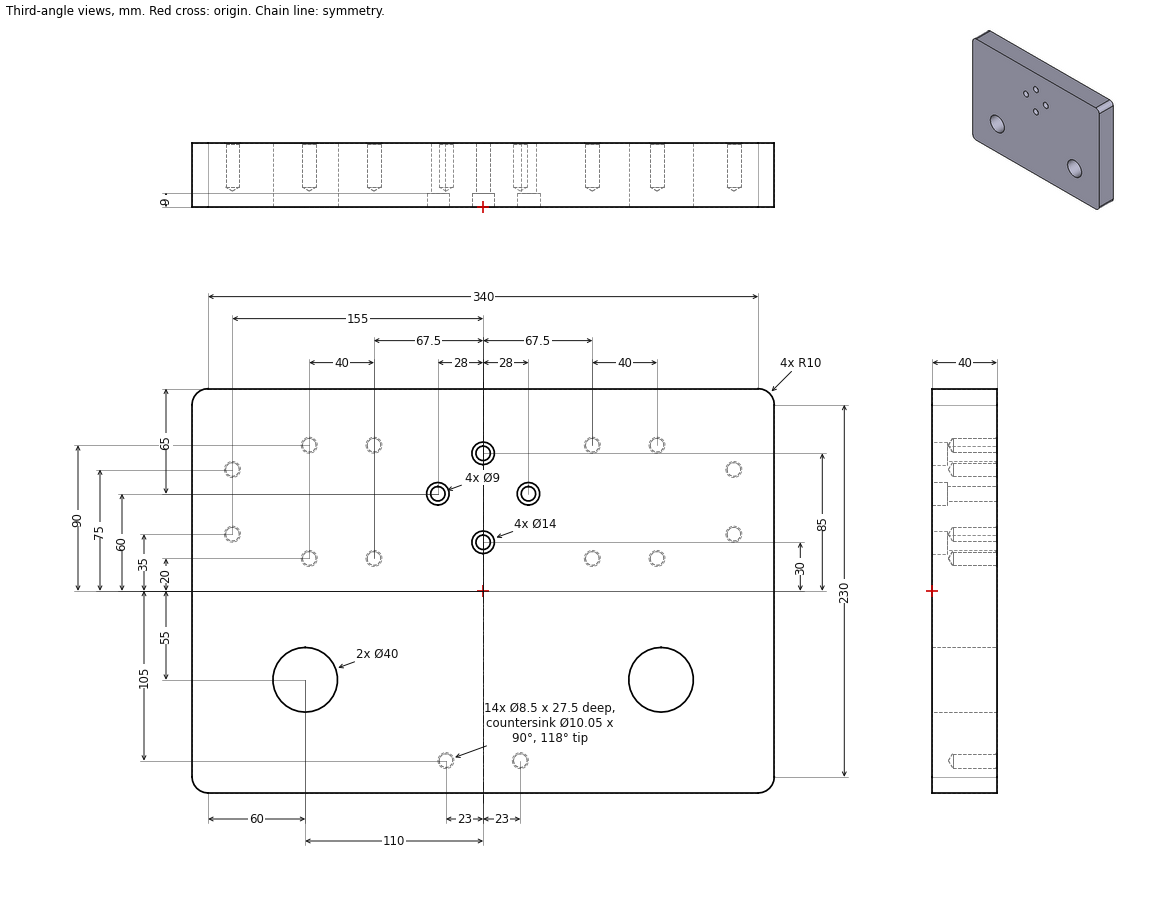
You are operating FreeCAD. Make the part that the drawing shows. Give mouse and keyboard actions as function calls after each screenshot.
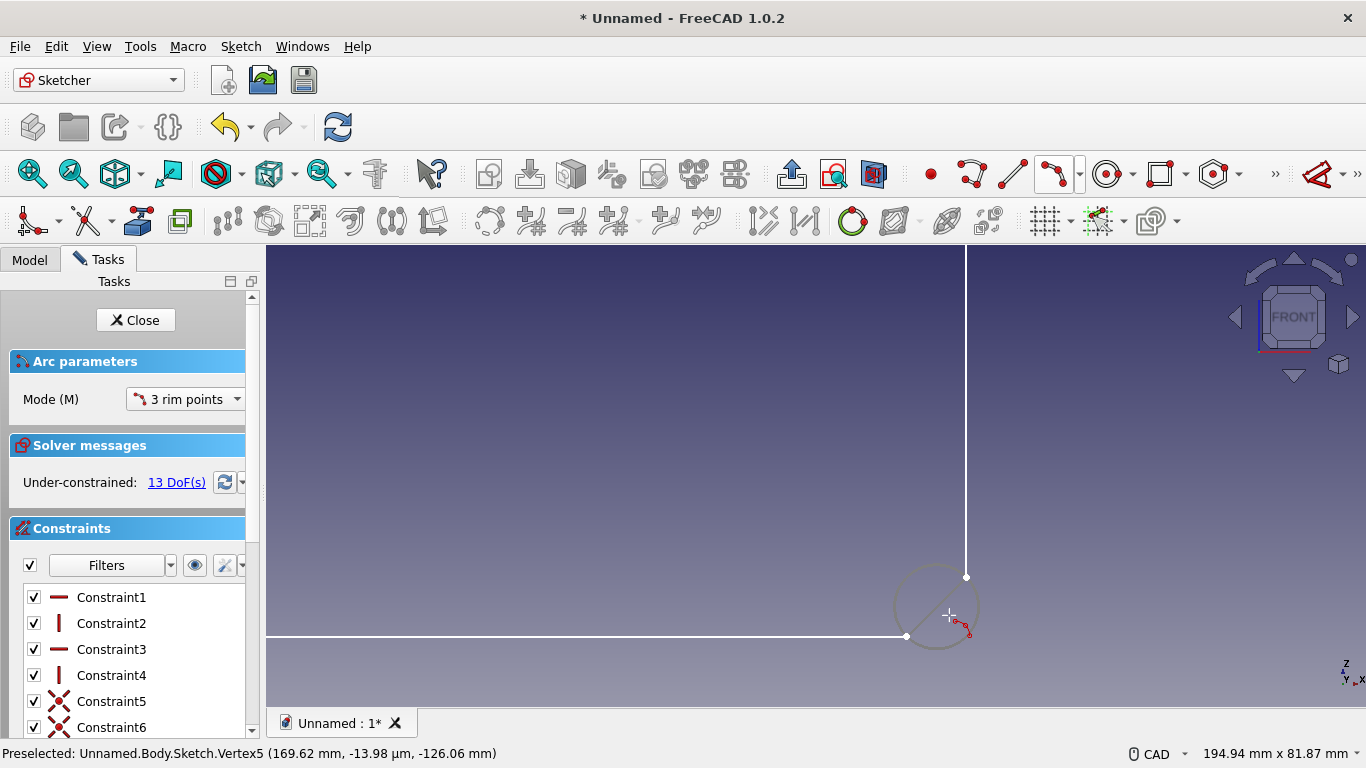
click(949, 614)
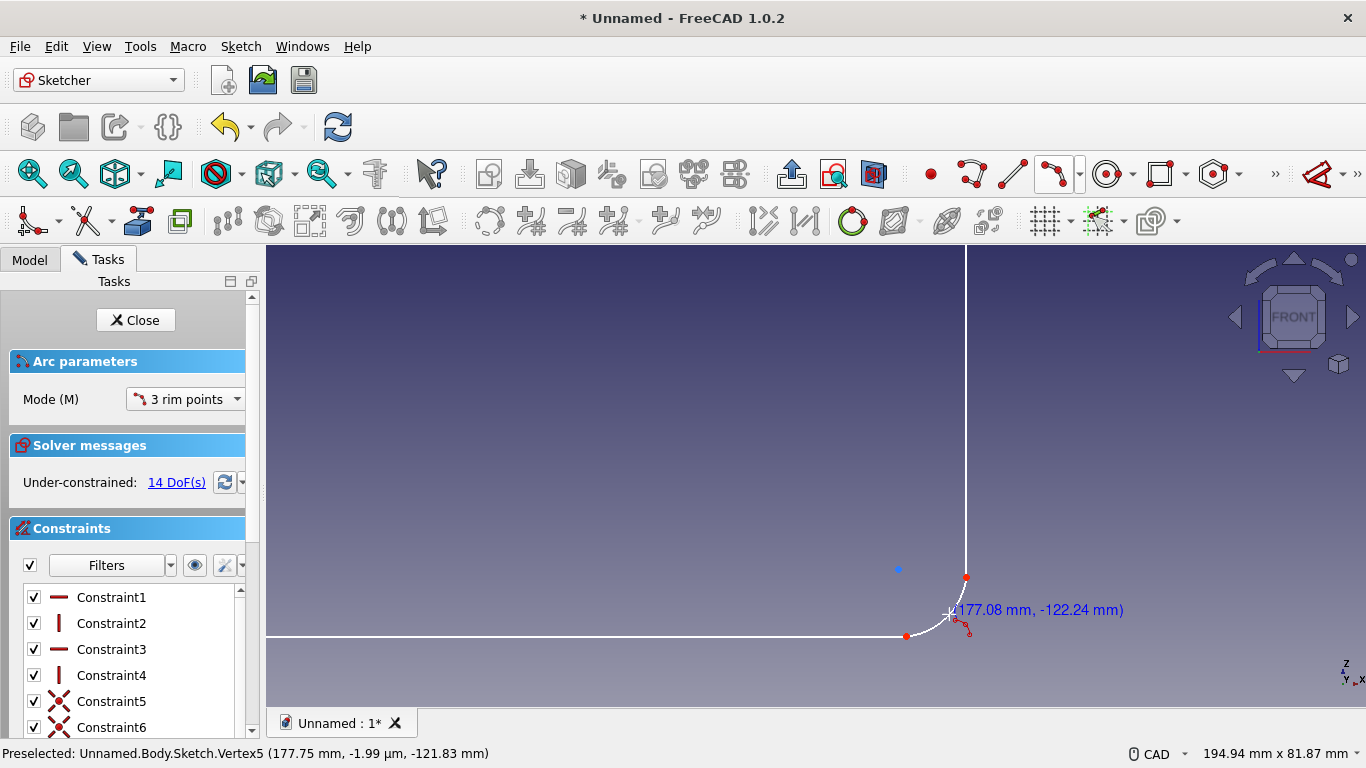
scroll(949, 615, down, 8)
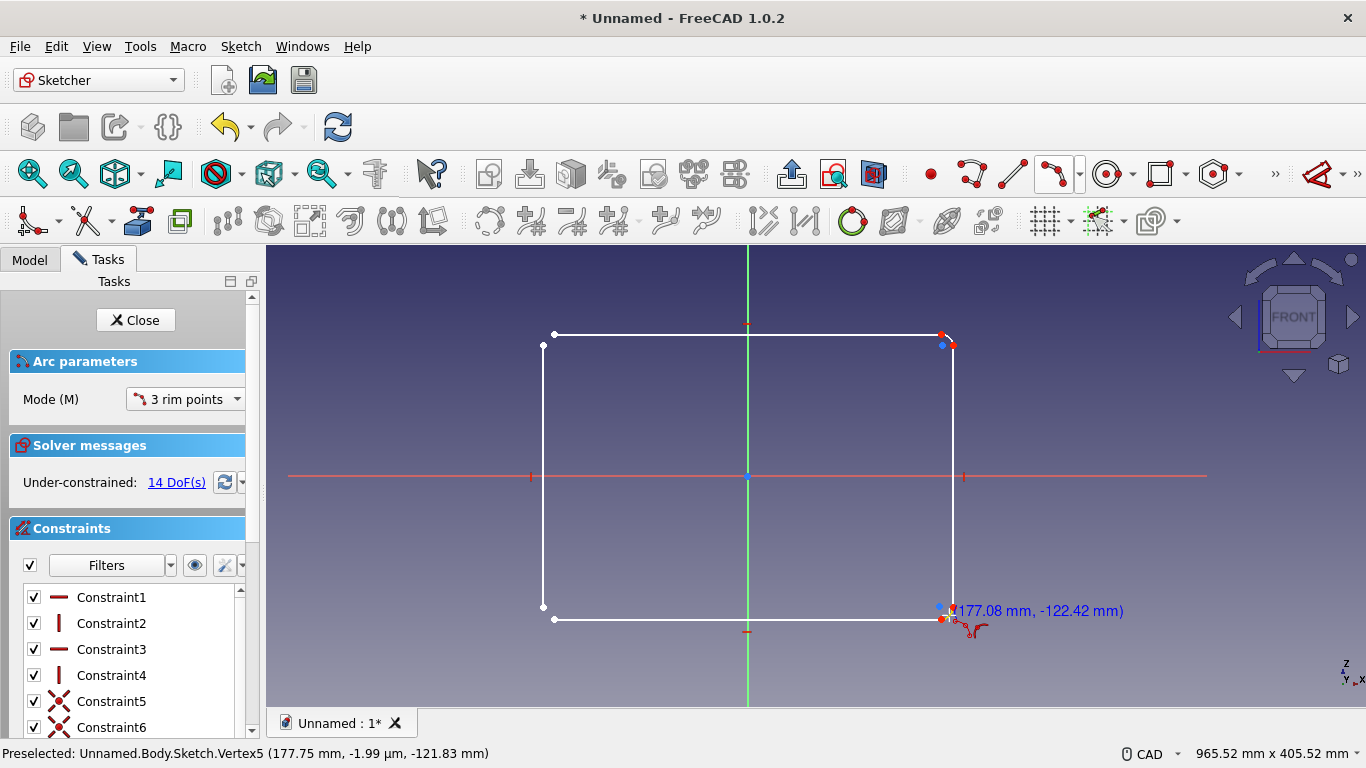
click(554, 620)
click(543, 608)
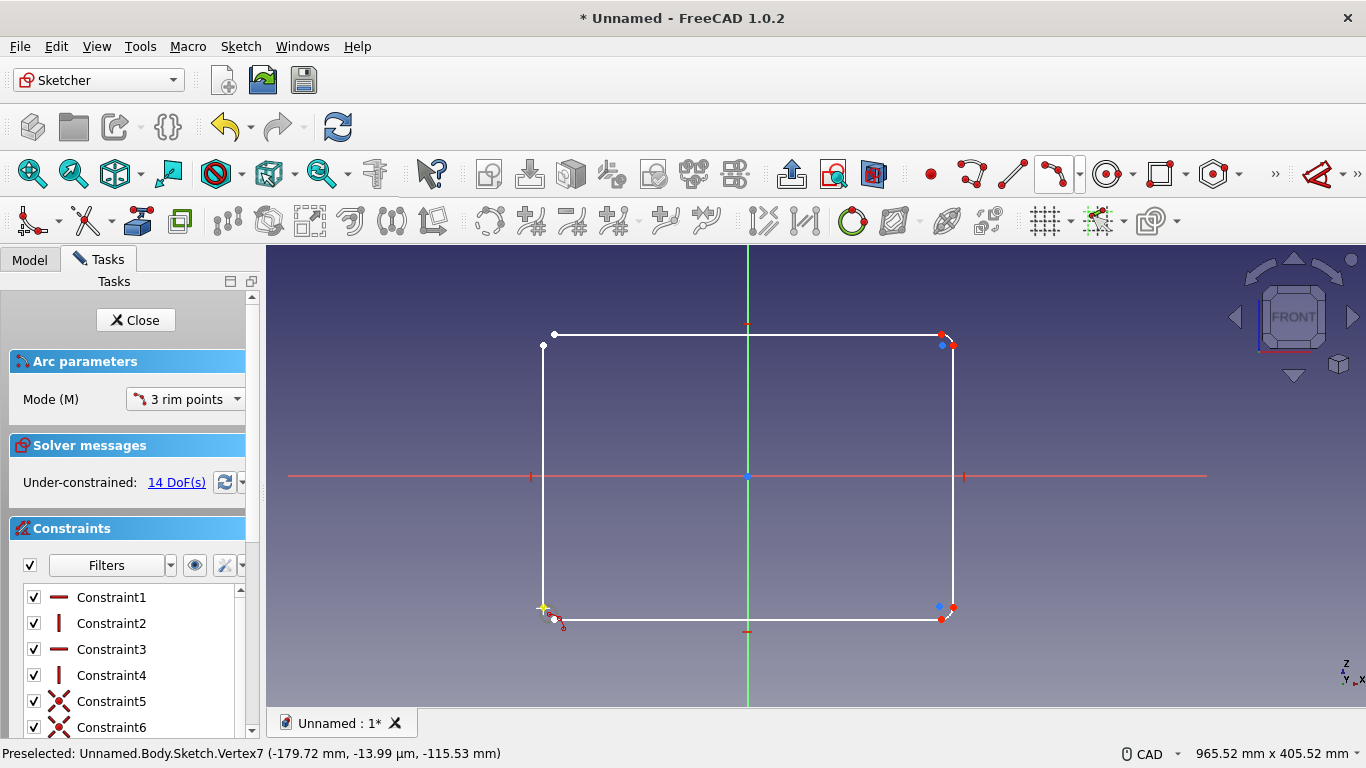
scroll(546, 615, up, 8)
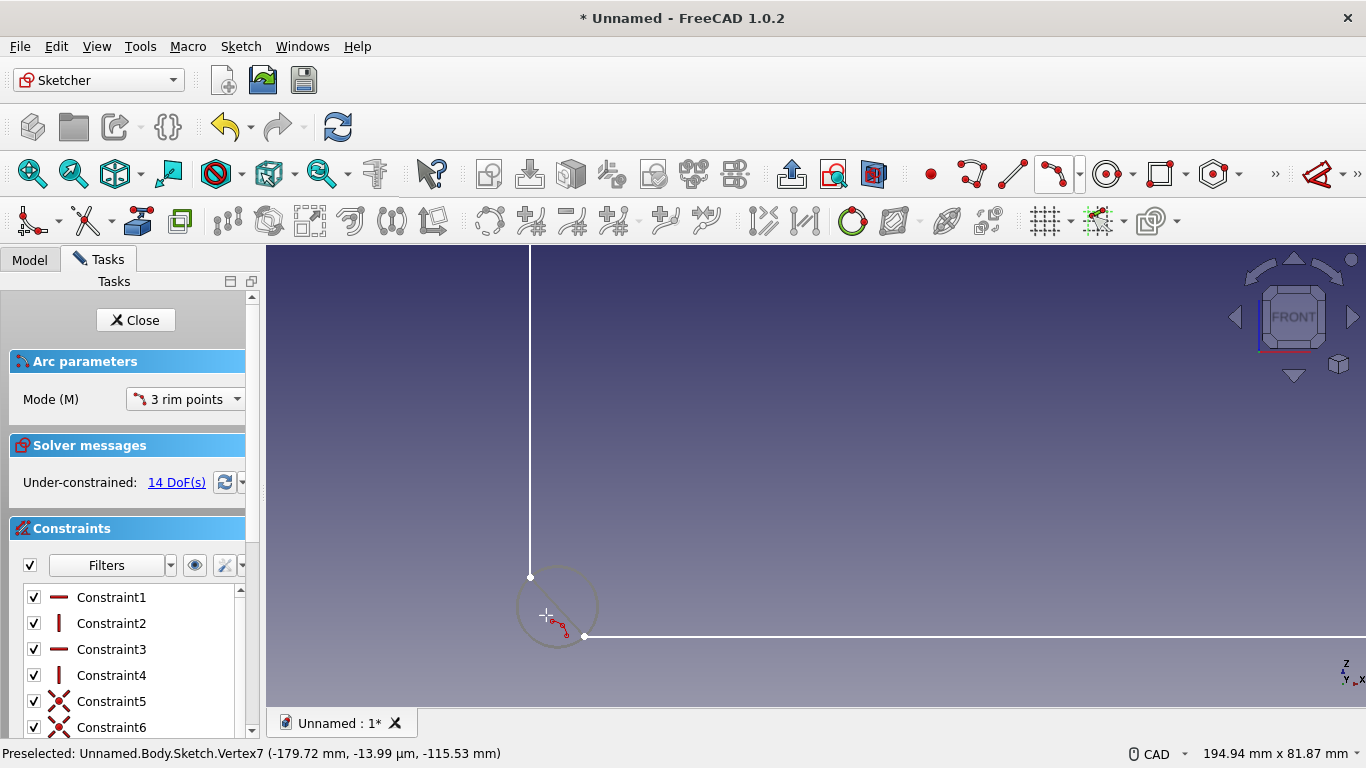
click(545, 614)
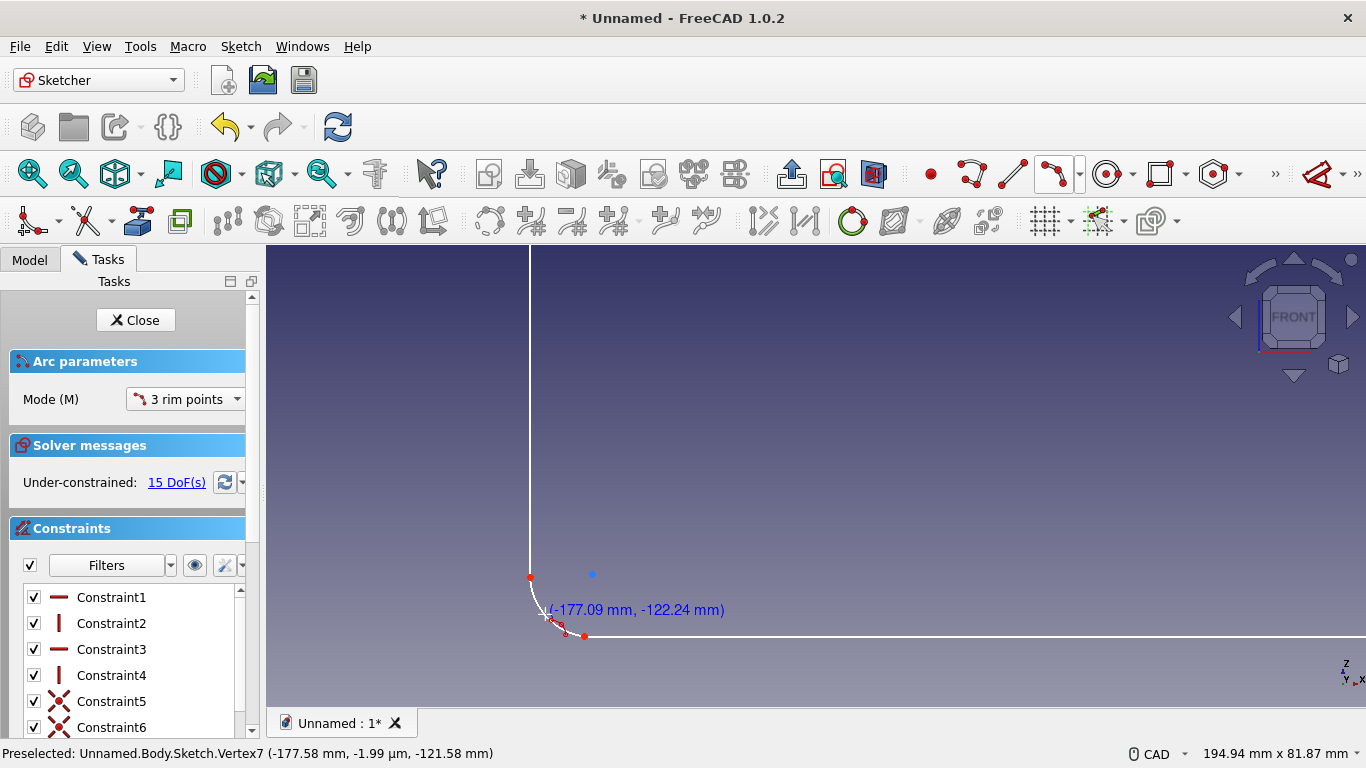
scroll(546, 615, down, 8)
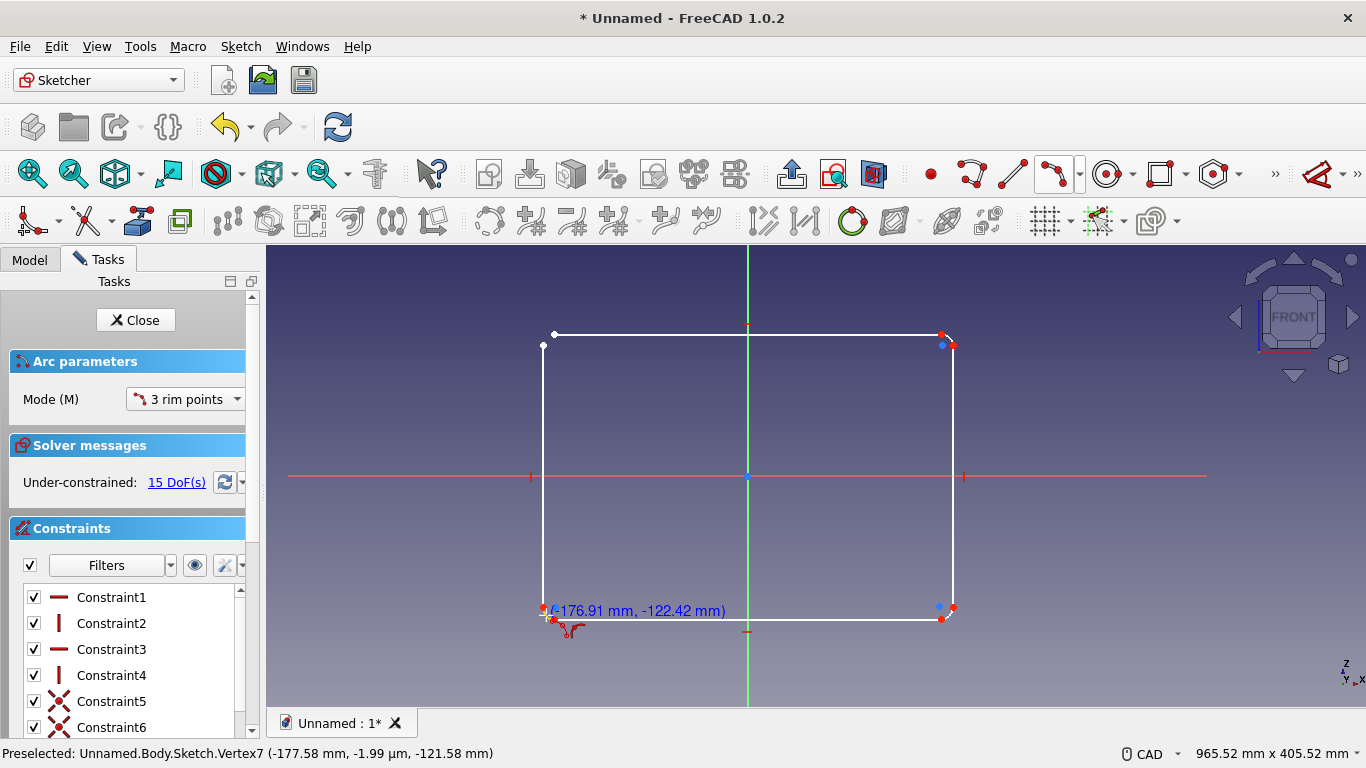
click(543, 346)
click(554, 335)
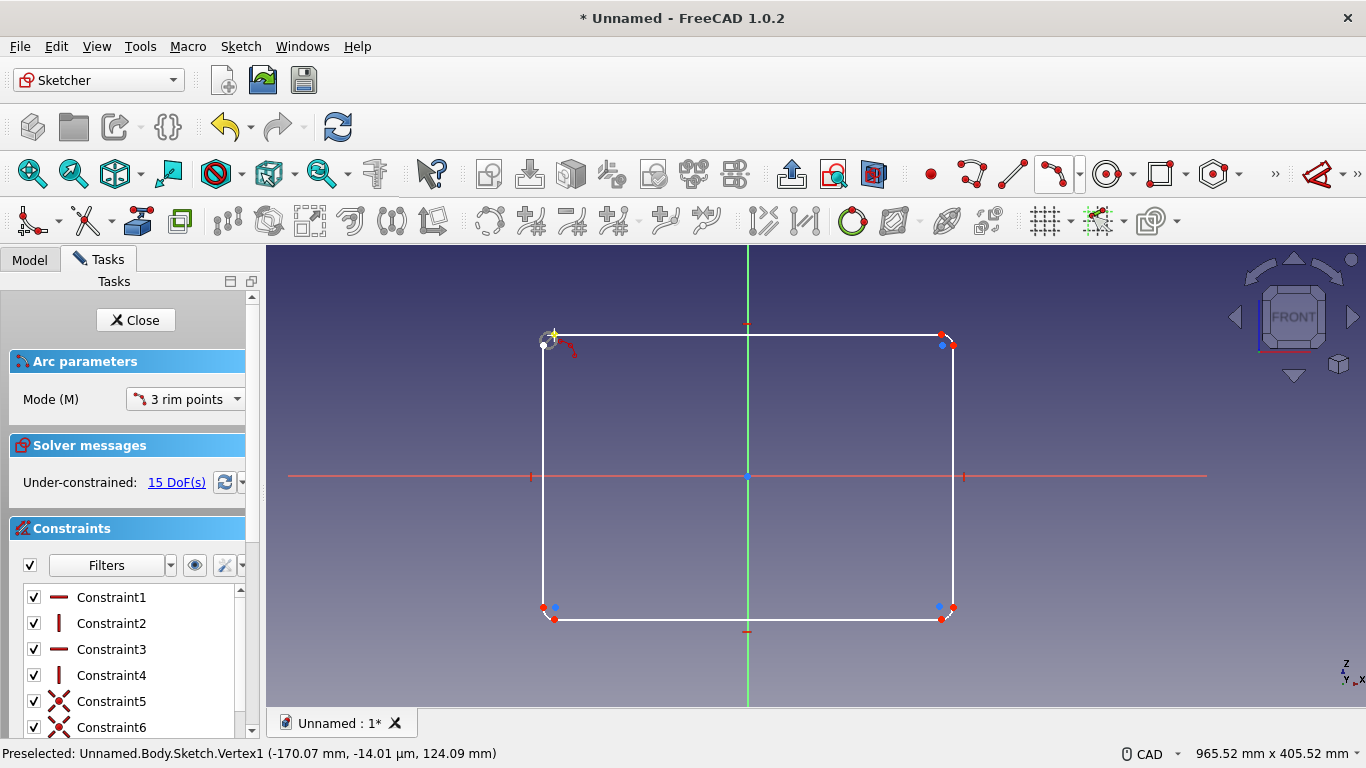
scroll(546, 337, up, 8)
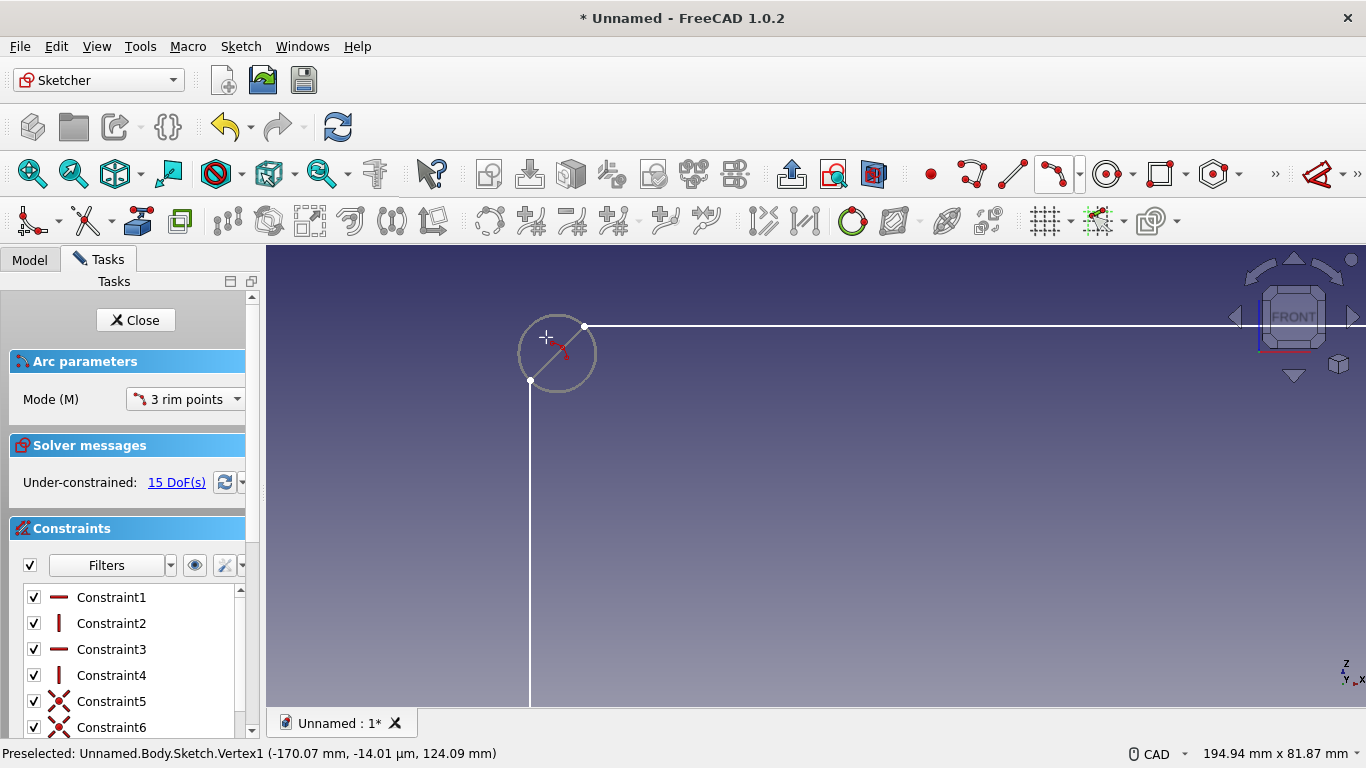
click(545, 338)